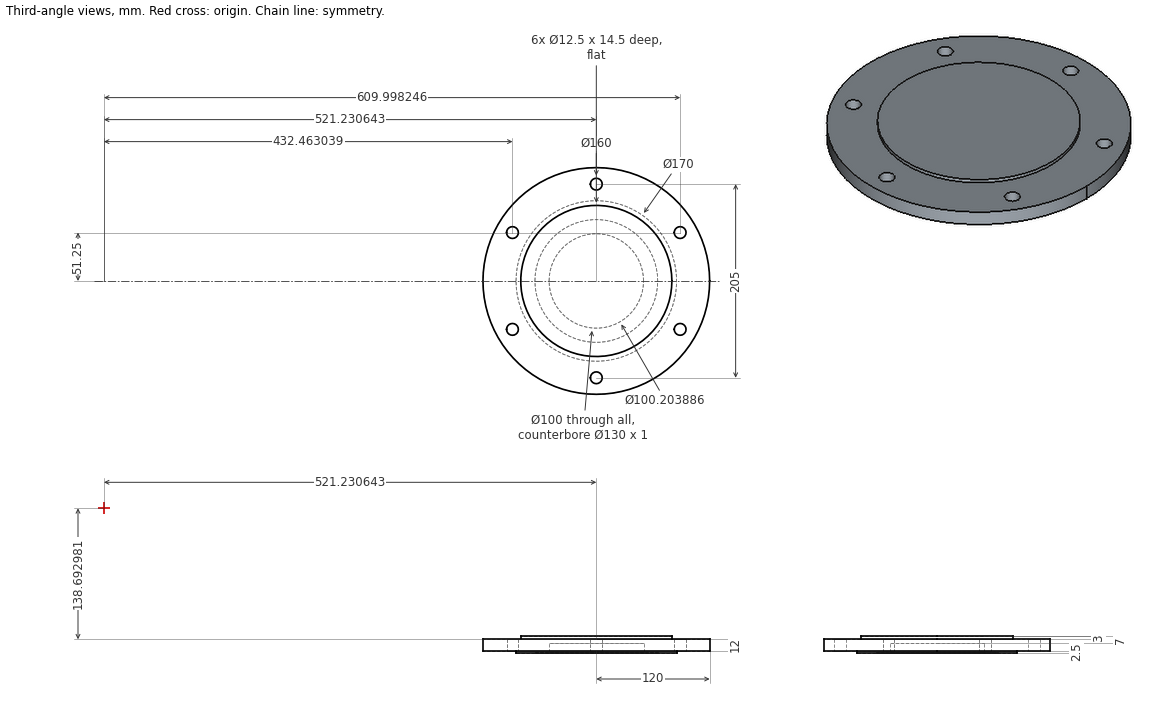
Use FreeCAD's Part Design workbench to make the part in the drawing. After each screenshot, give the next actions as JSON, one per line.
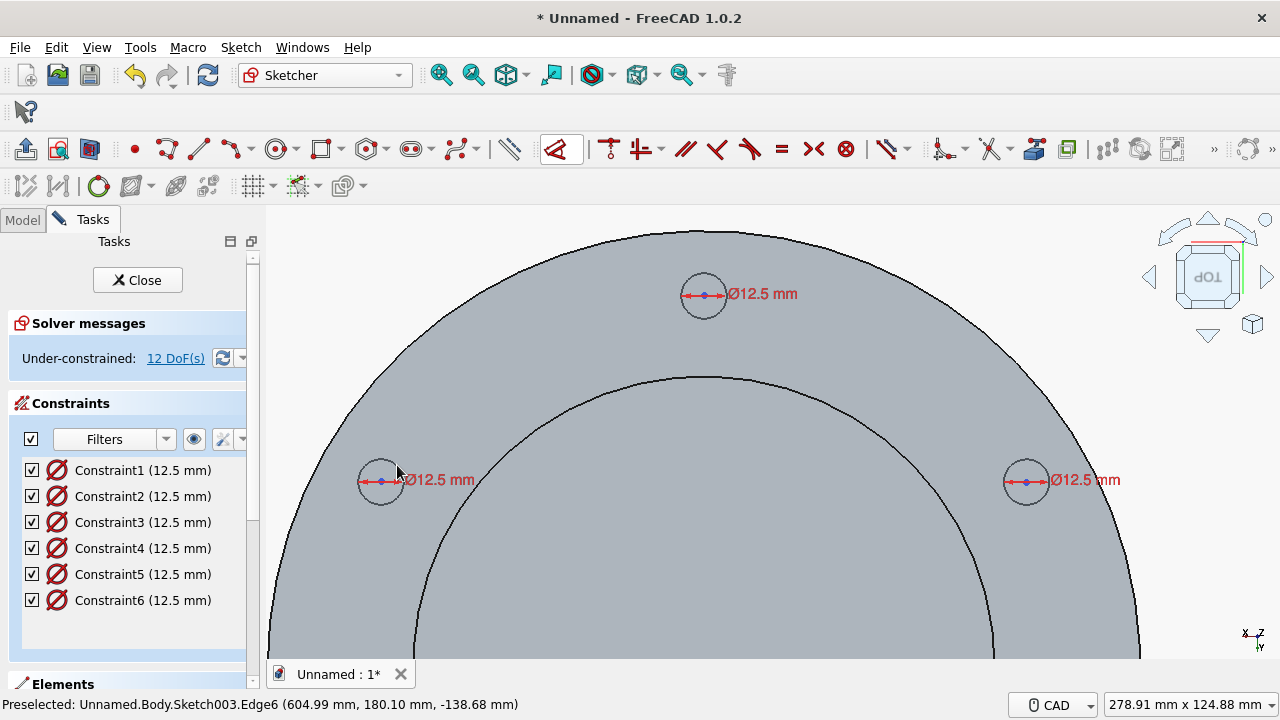
{"action": "scroll", "coordinate": [705, 295], "scroll_direction": "down", "scroll_amount": 5}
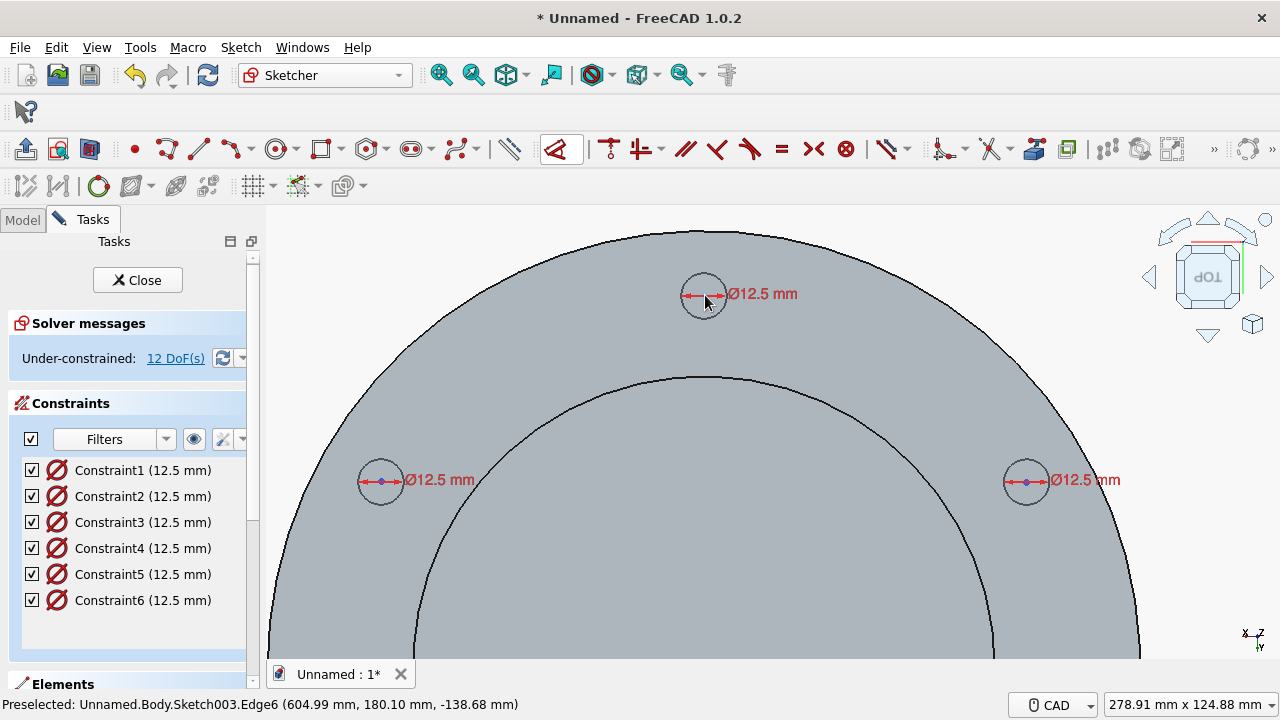
{"action": "left_click", "coordinate": [824, 501]}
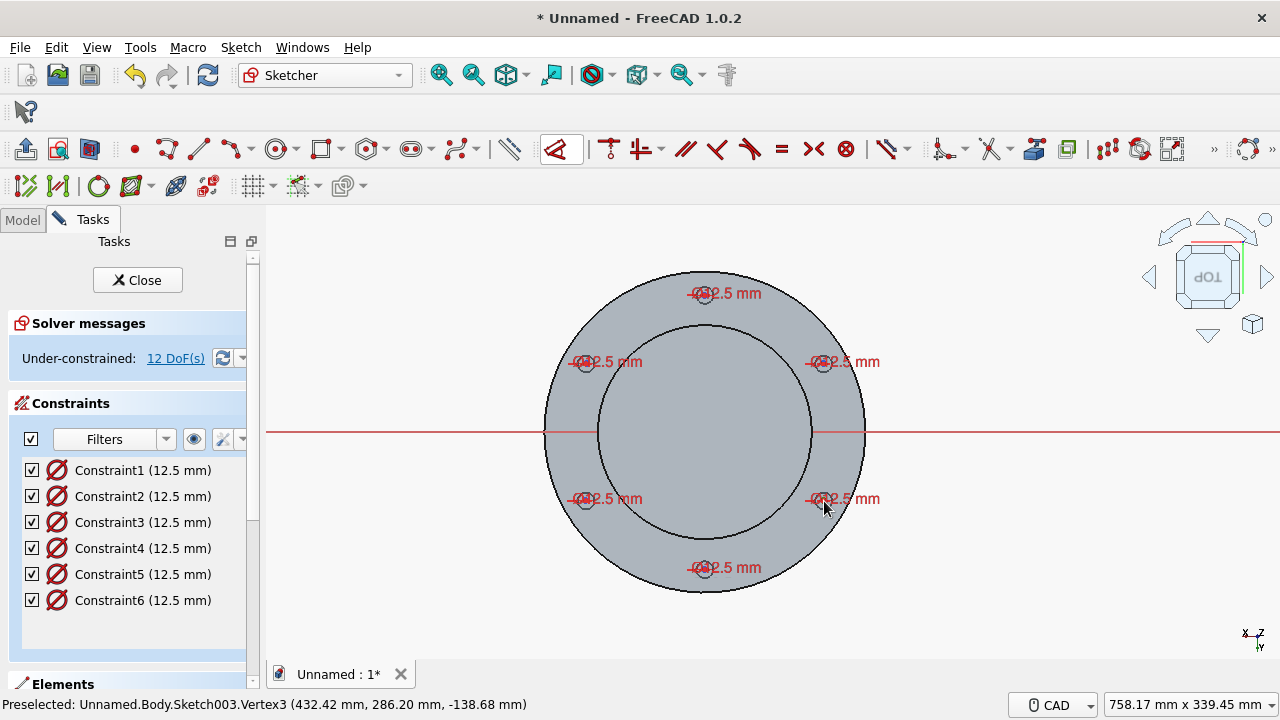
{"action": "left_click", "coordinate": [824, 364]}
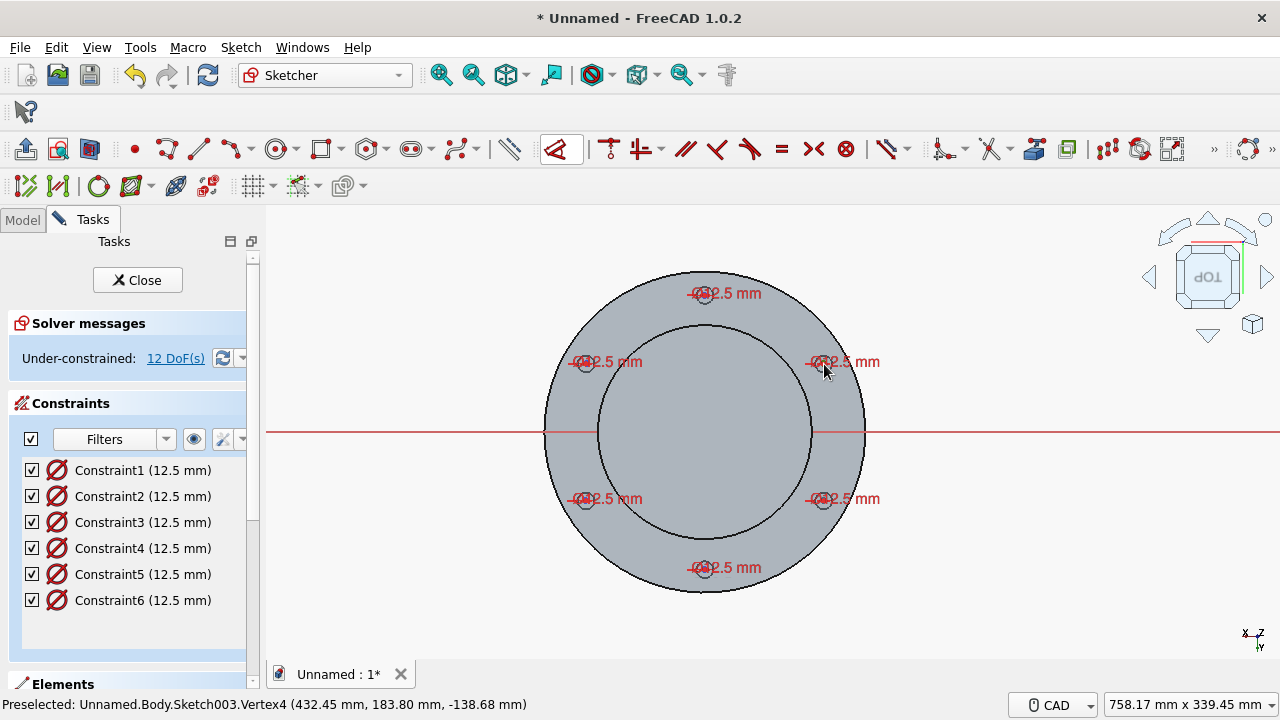
{"action": "left_click", "coordinate": [353, 432]}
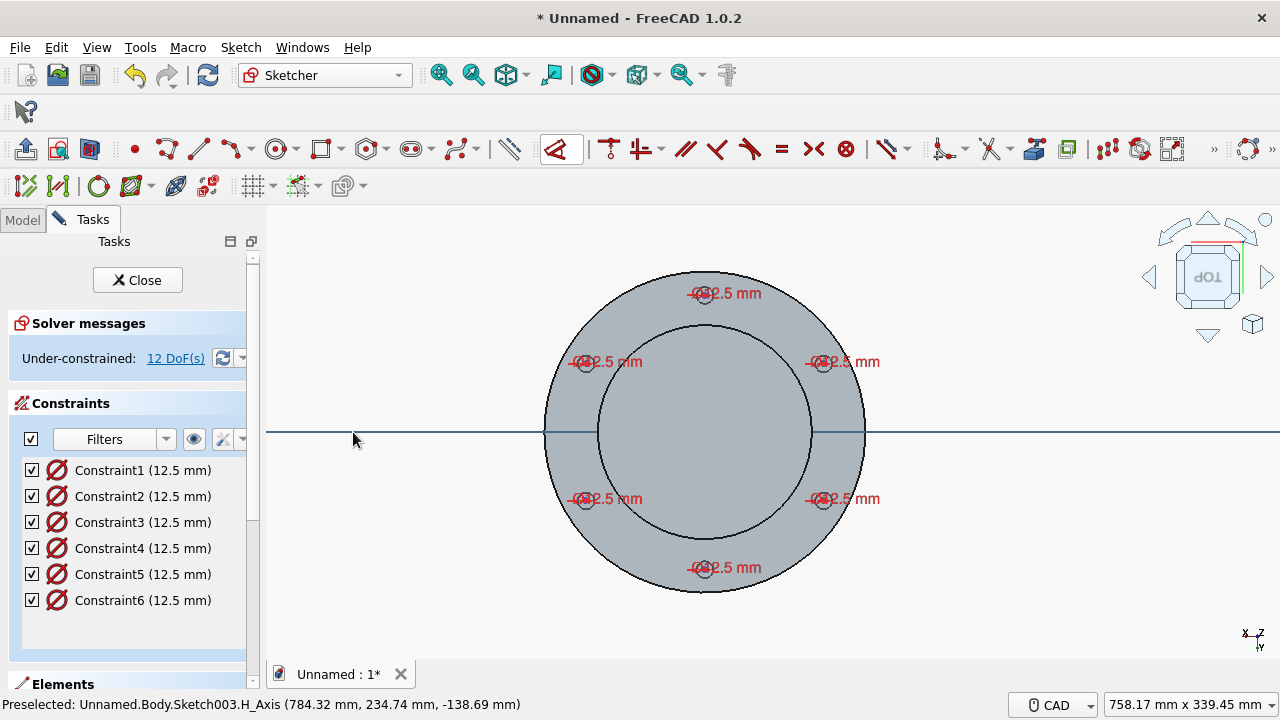
{"action": "key", "text": "s"}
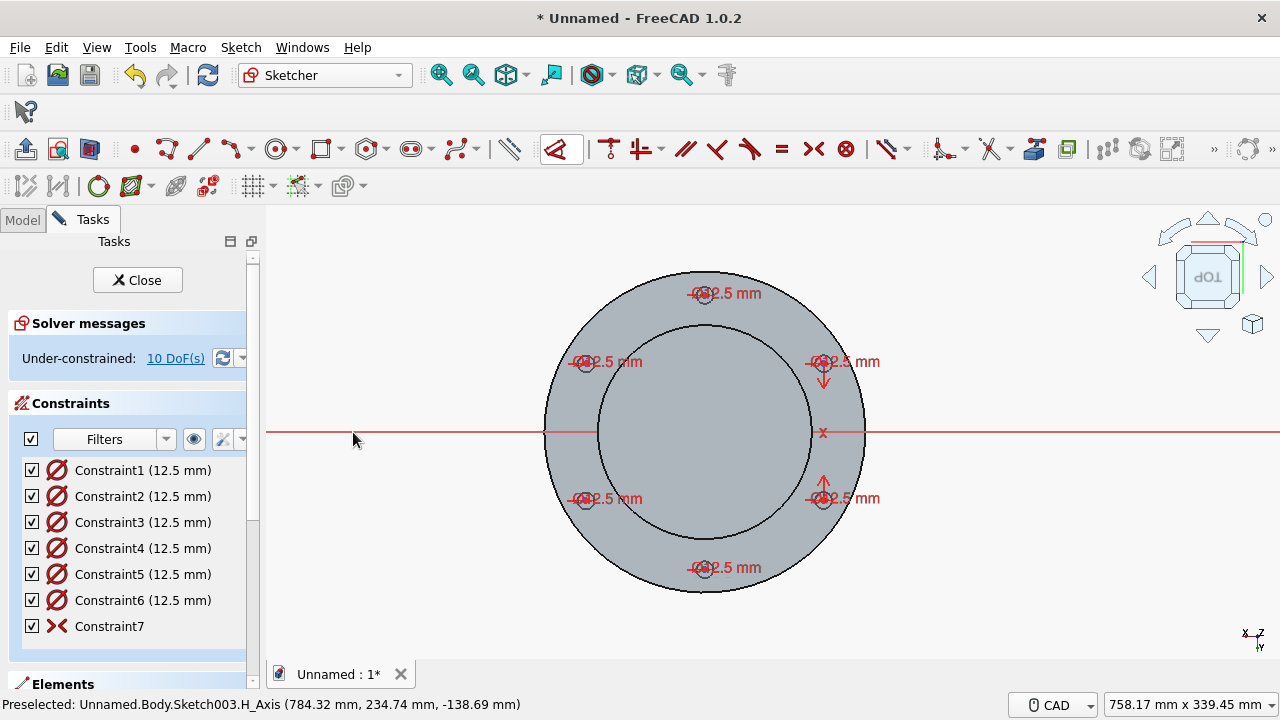
{"action": "left_click", "coordinate": [705, 570]}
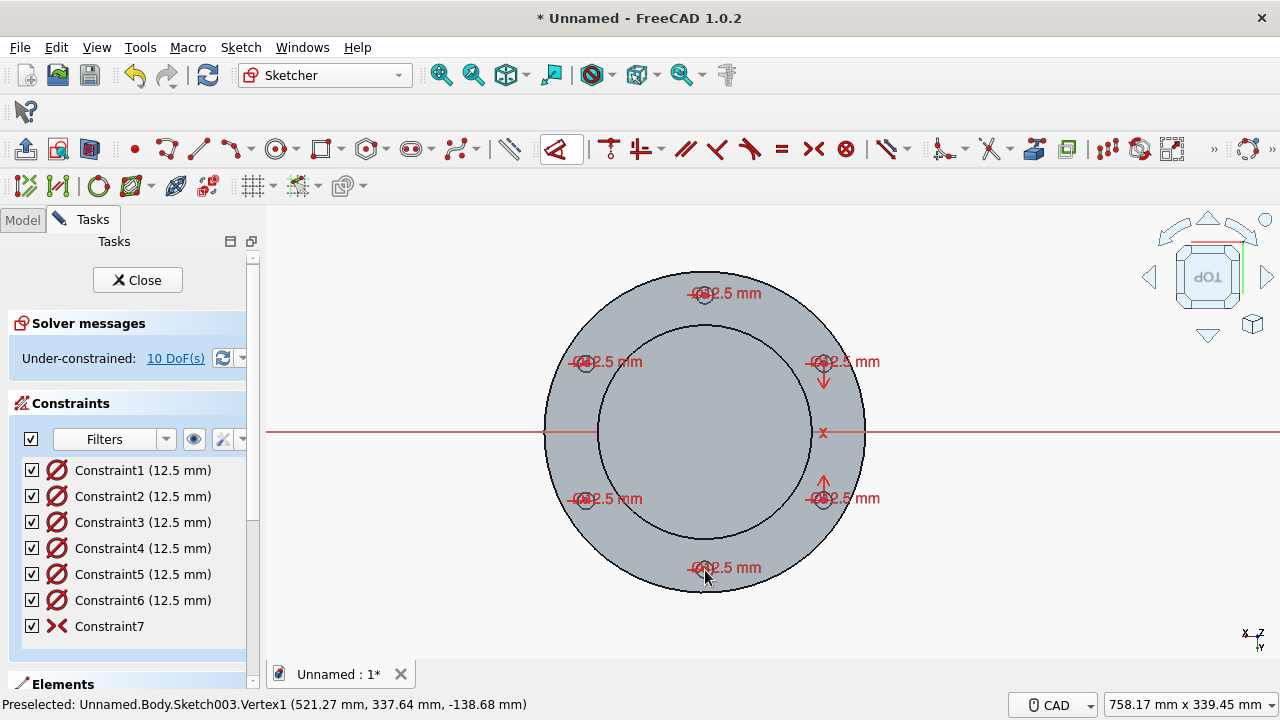
{"action": "left_click", "coordinate": [705, 295]}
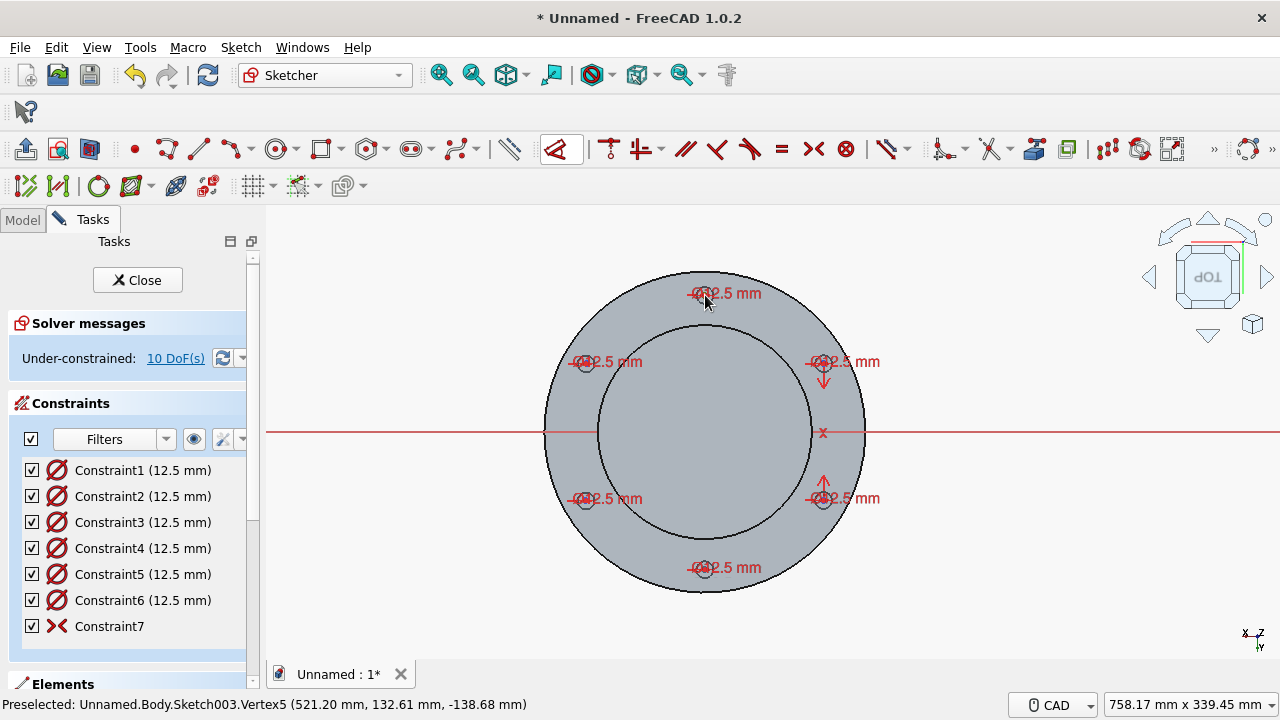
{"action": "left_click", "coordinate": [353, 432]}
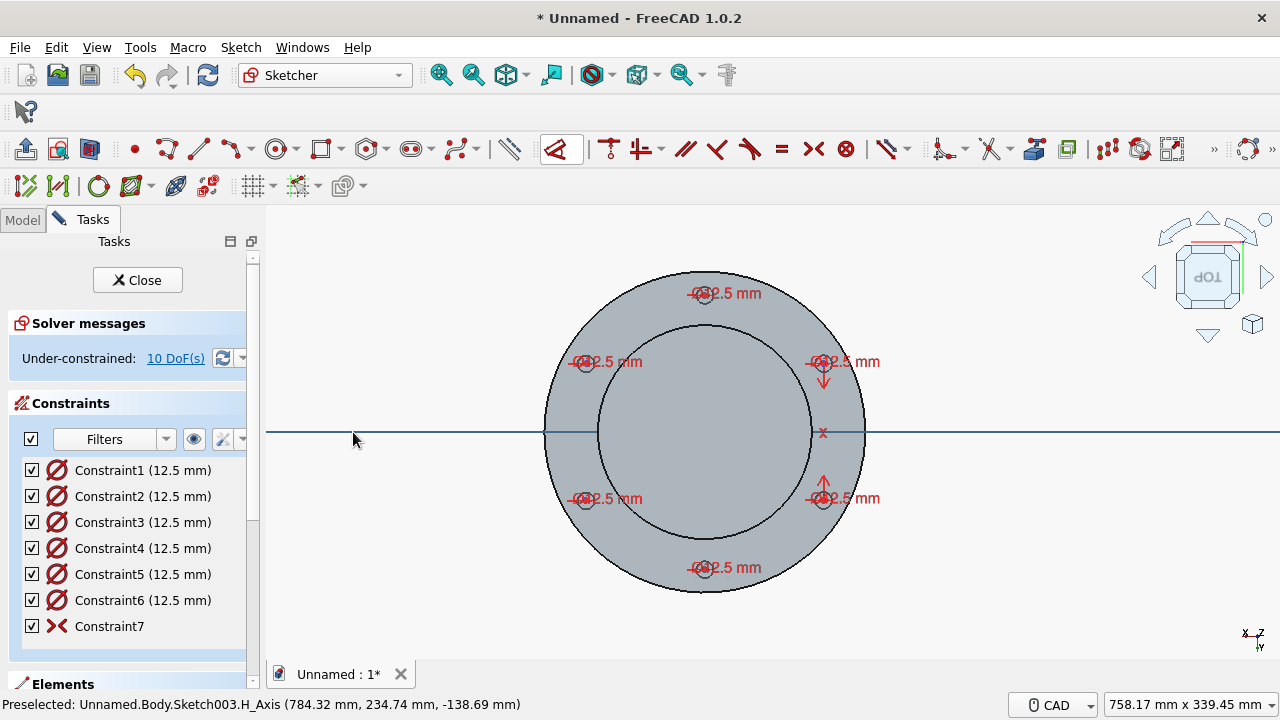
{"action": "key", "text": "s"}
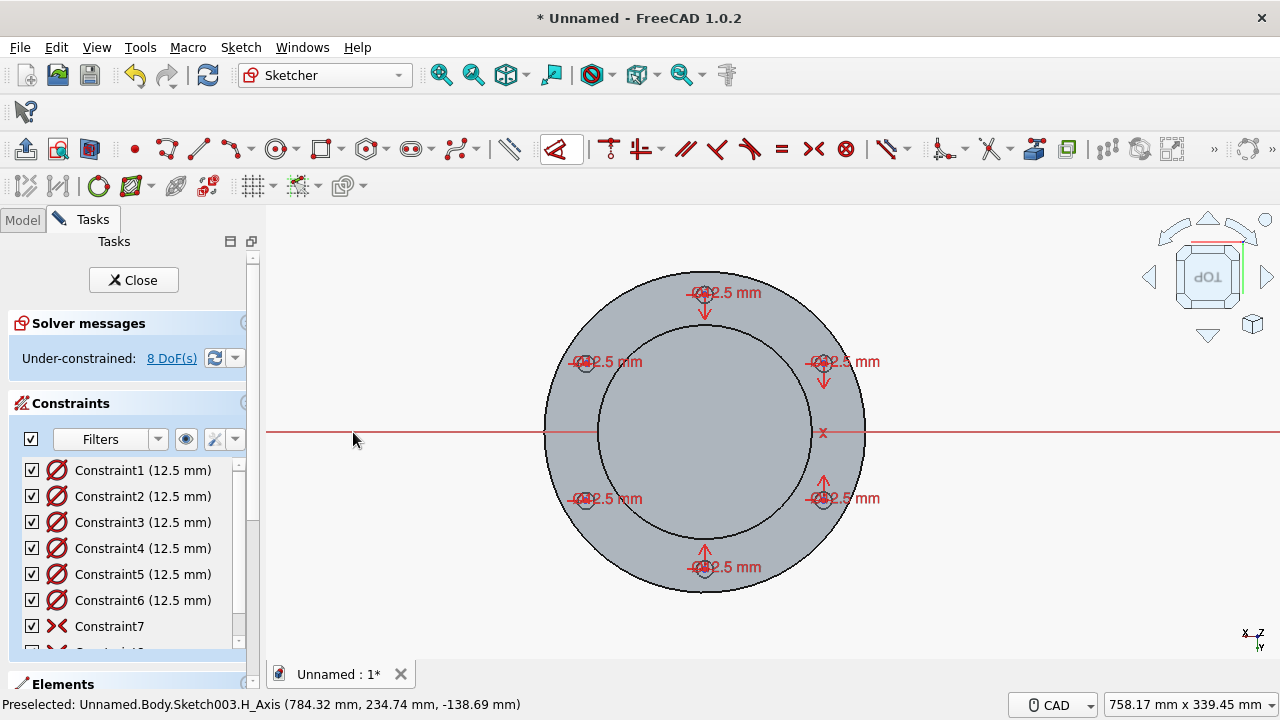
{"action": "left_click", "coordinate": [586, 501]}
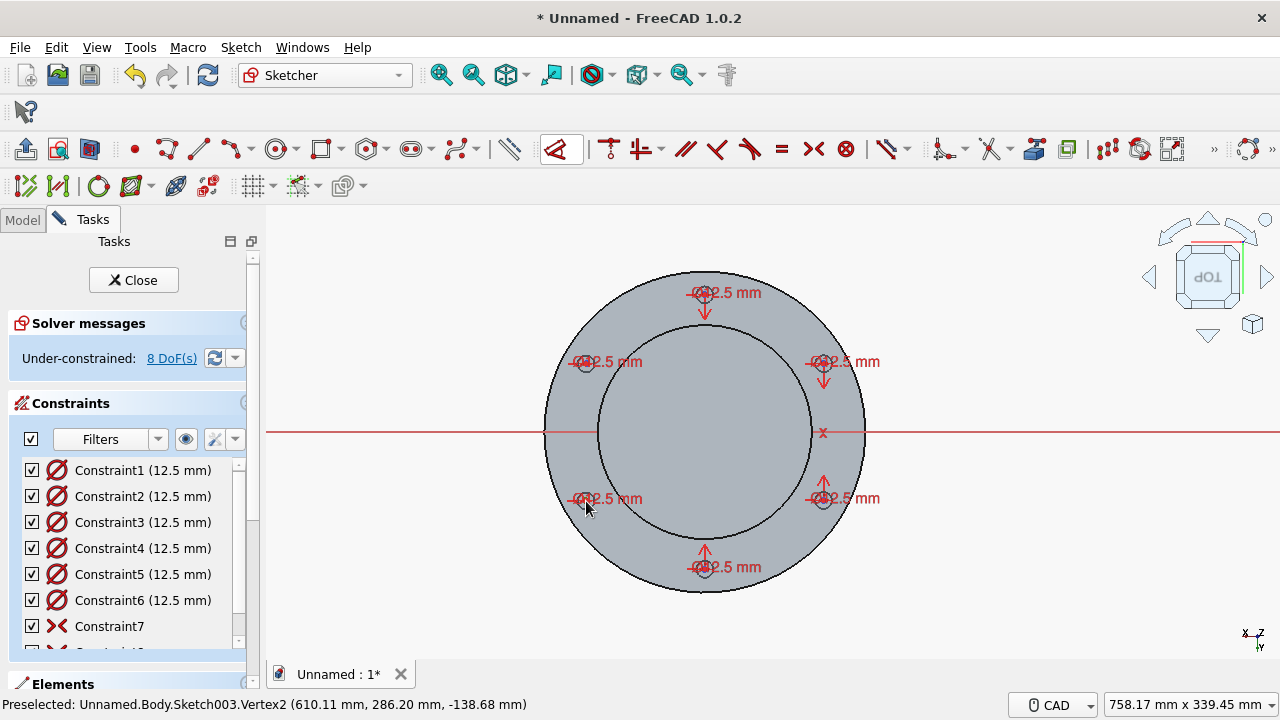
{"action": "left_click", "coordinate": [586, 364]}